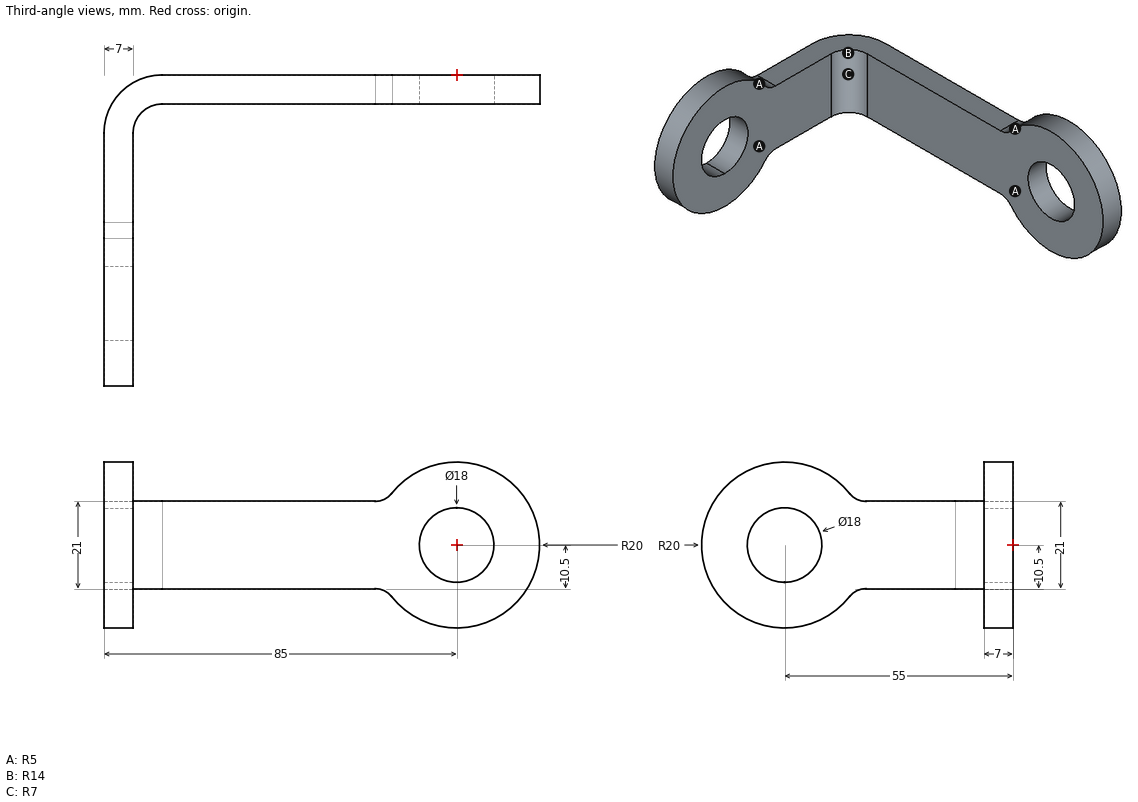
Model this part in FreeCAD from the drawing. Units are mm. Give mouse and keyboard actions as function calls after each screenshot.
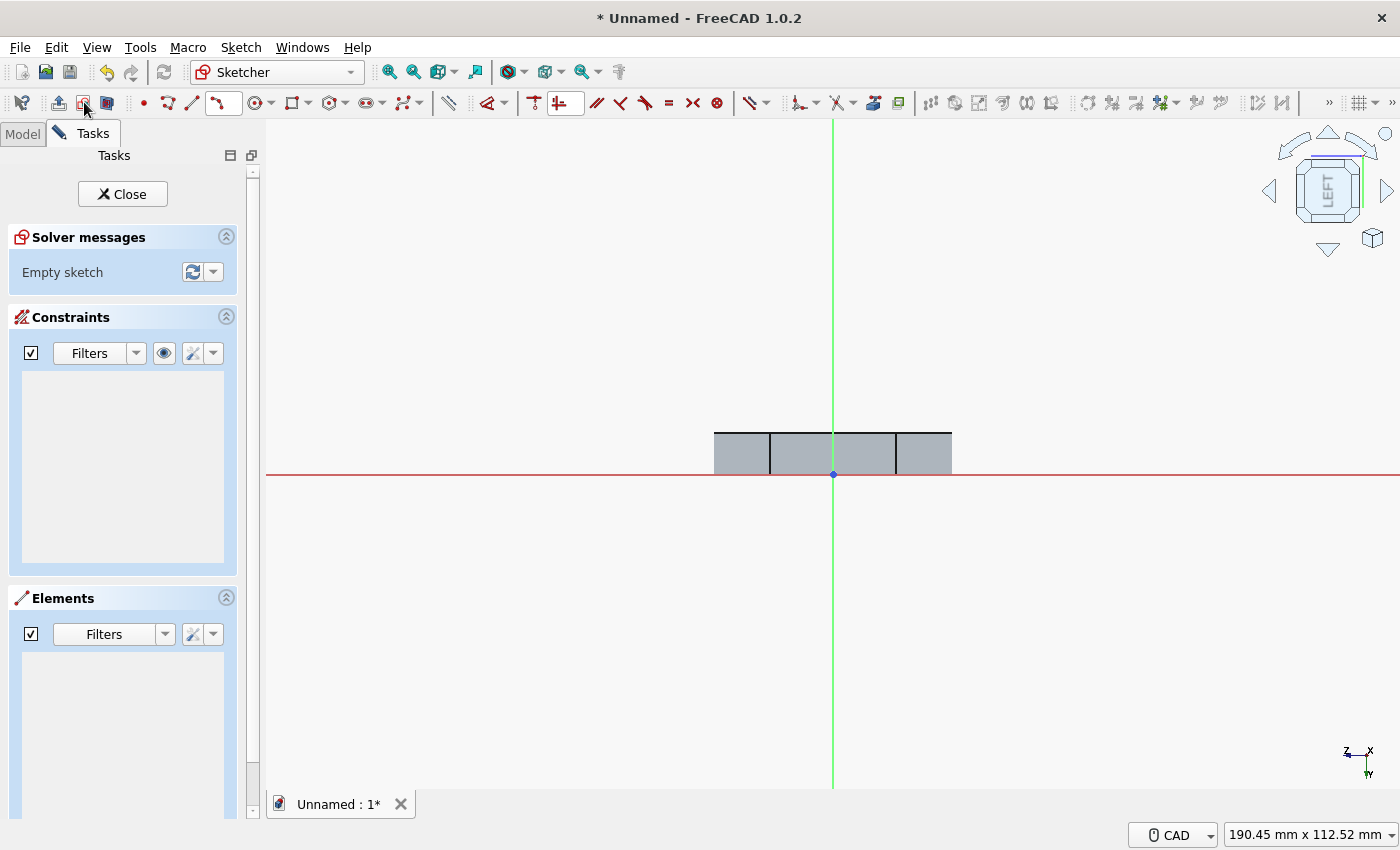
scroll(625, 761, down, 2)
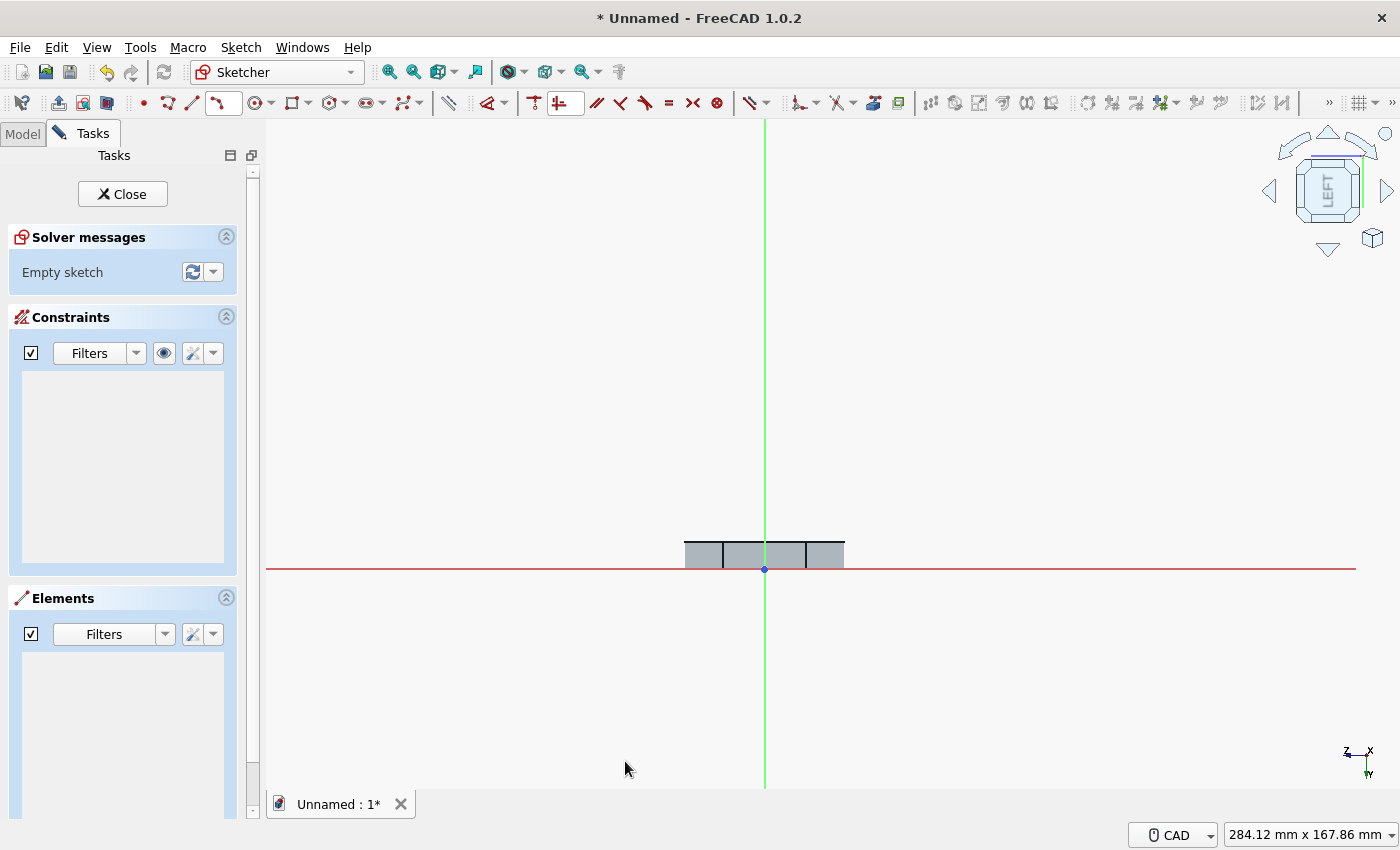
scroll(765, 350, up, 2)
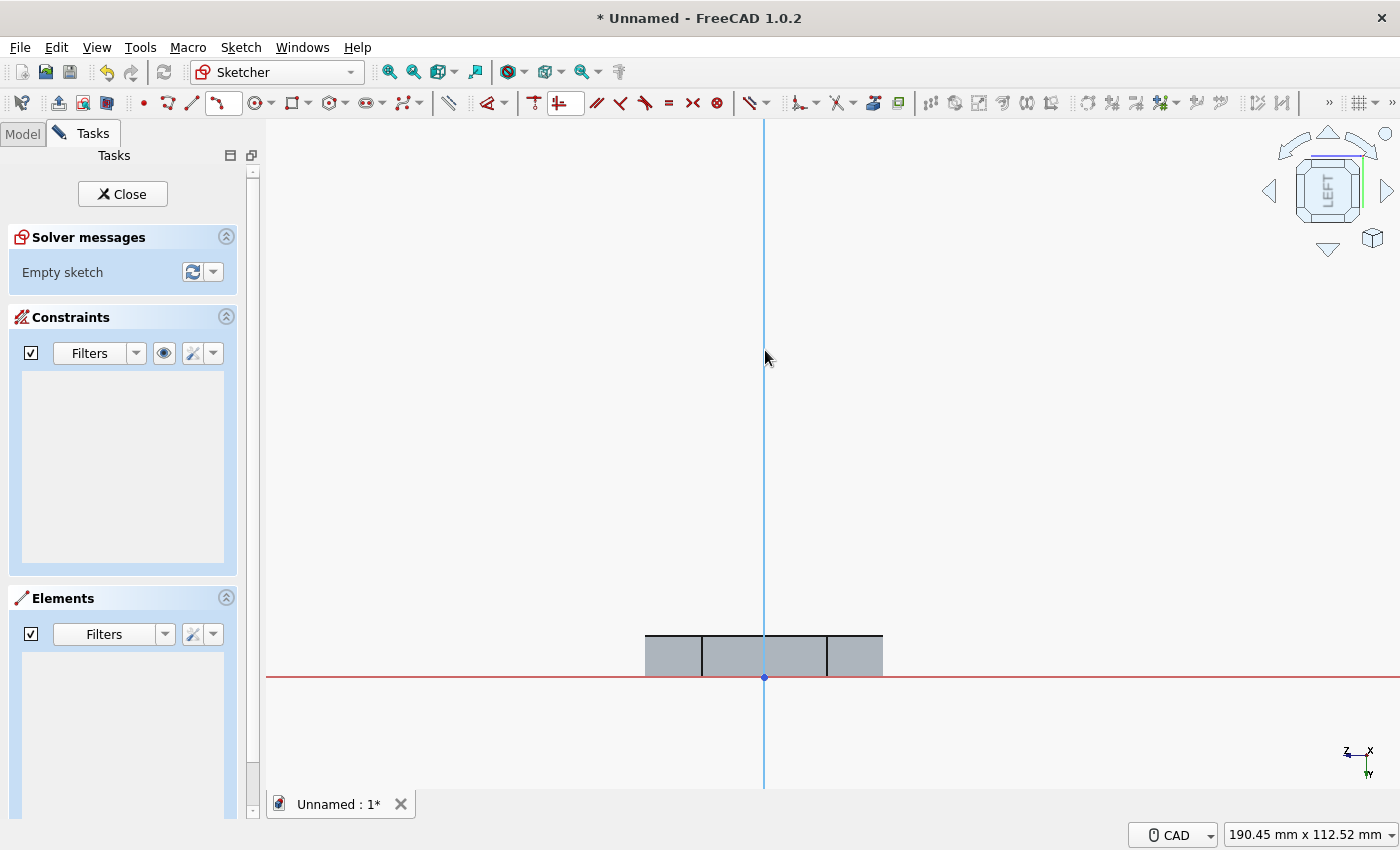
click(168, 104)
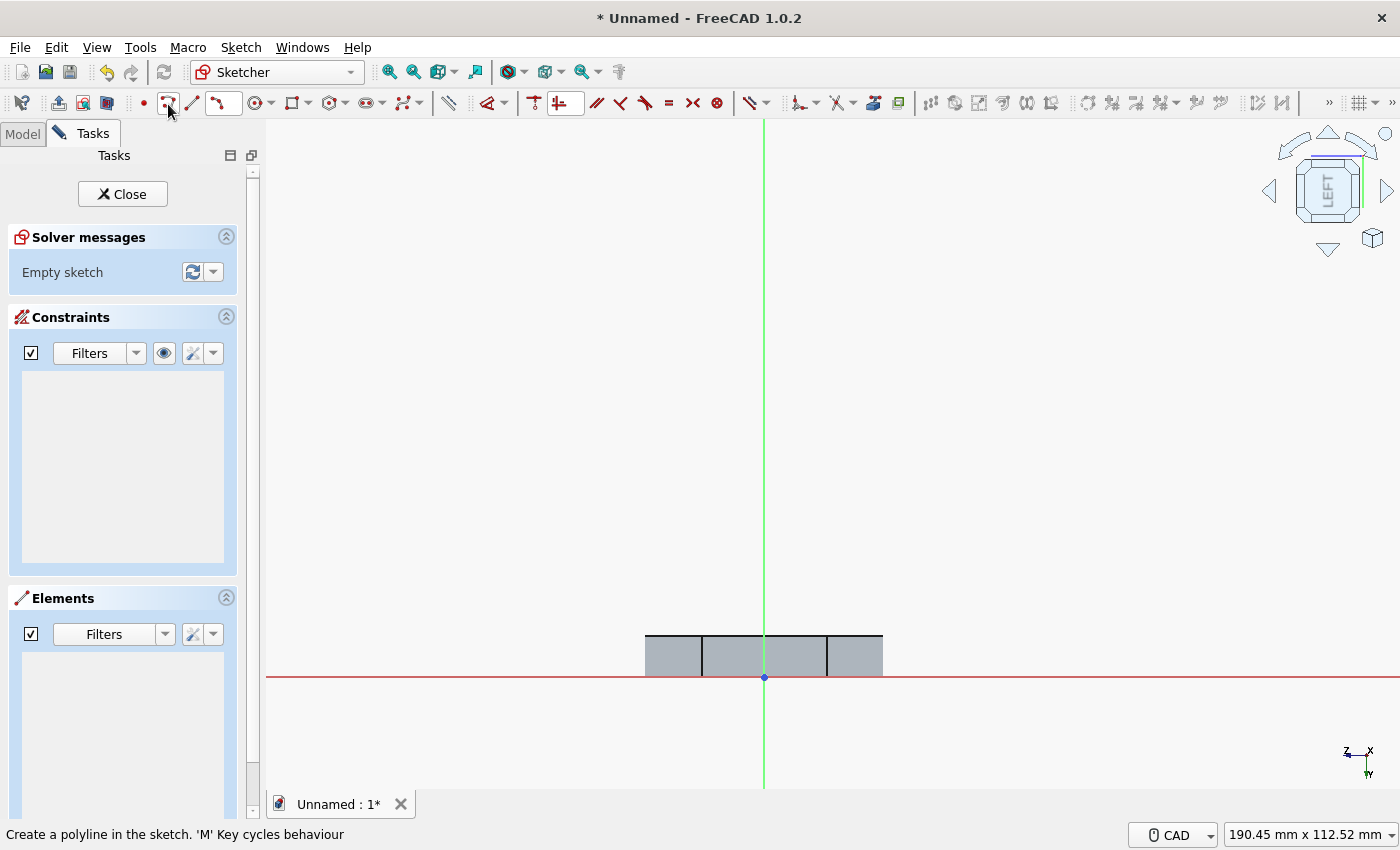
click(827, 451)
click(827, 677)
click(702, 668)
click(702, 451)
right_click(702, 451)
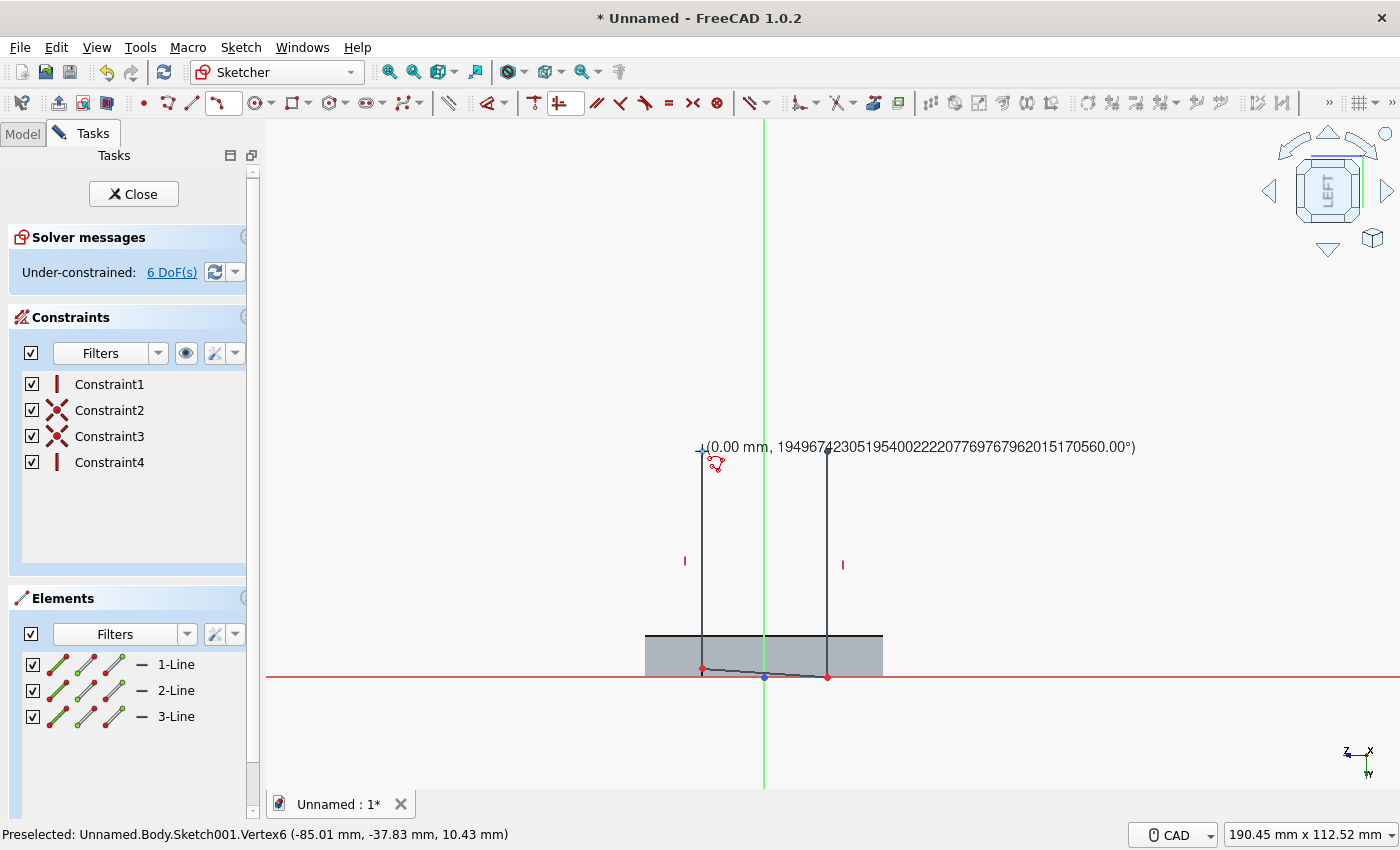
click(218, 104)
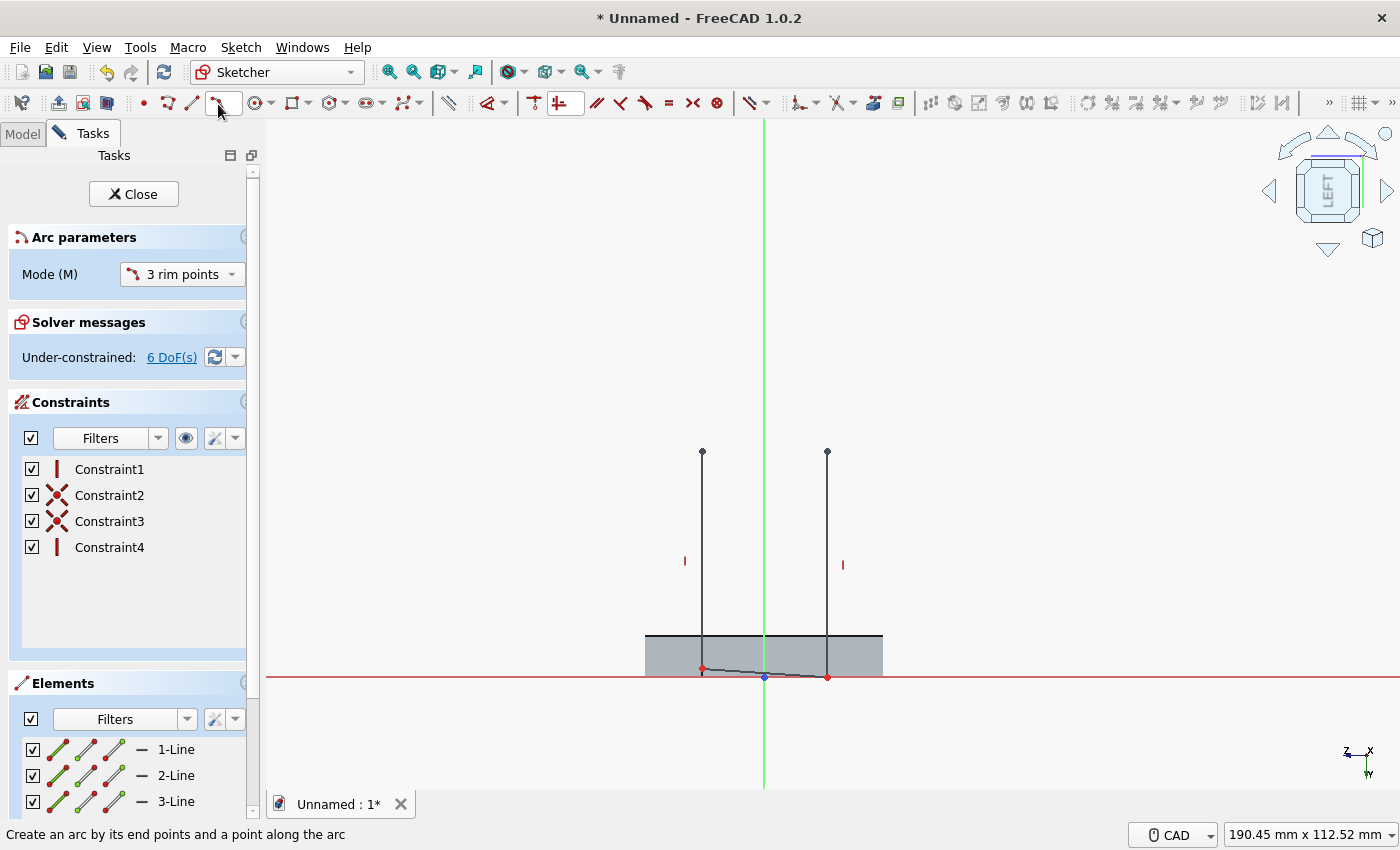
click(702, 452)
click(827, 452)
click(823, 246)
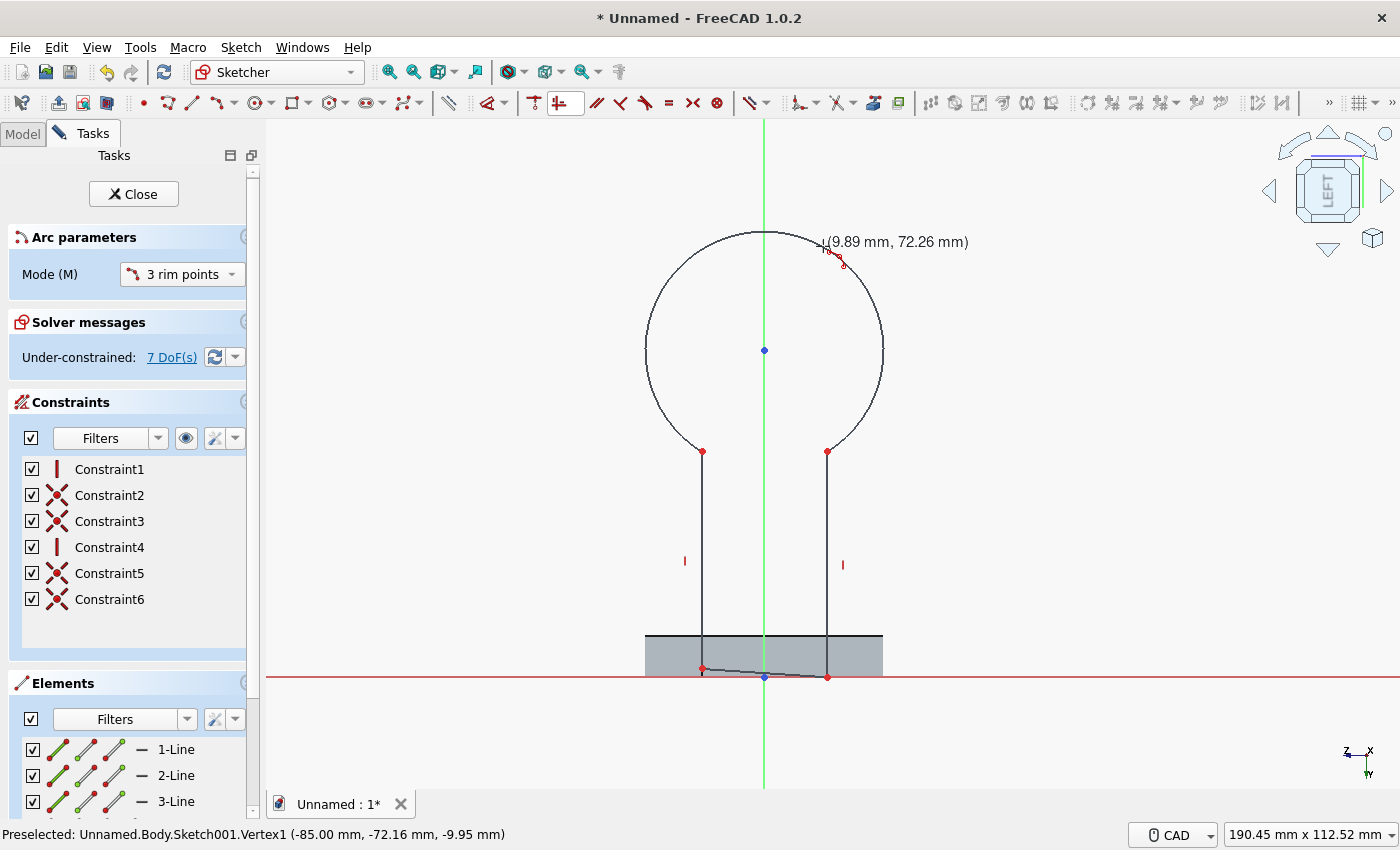
click(256, 104)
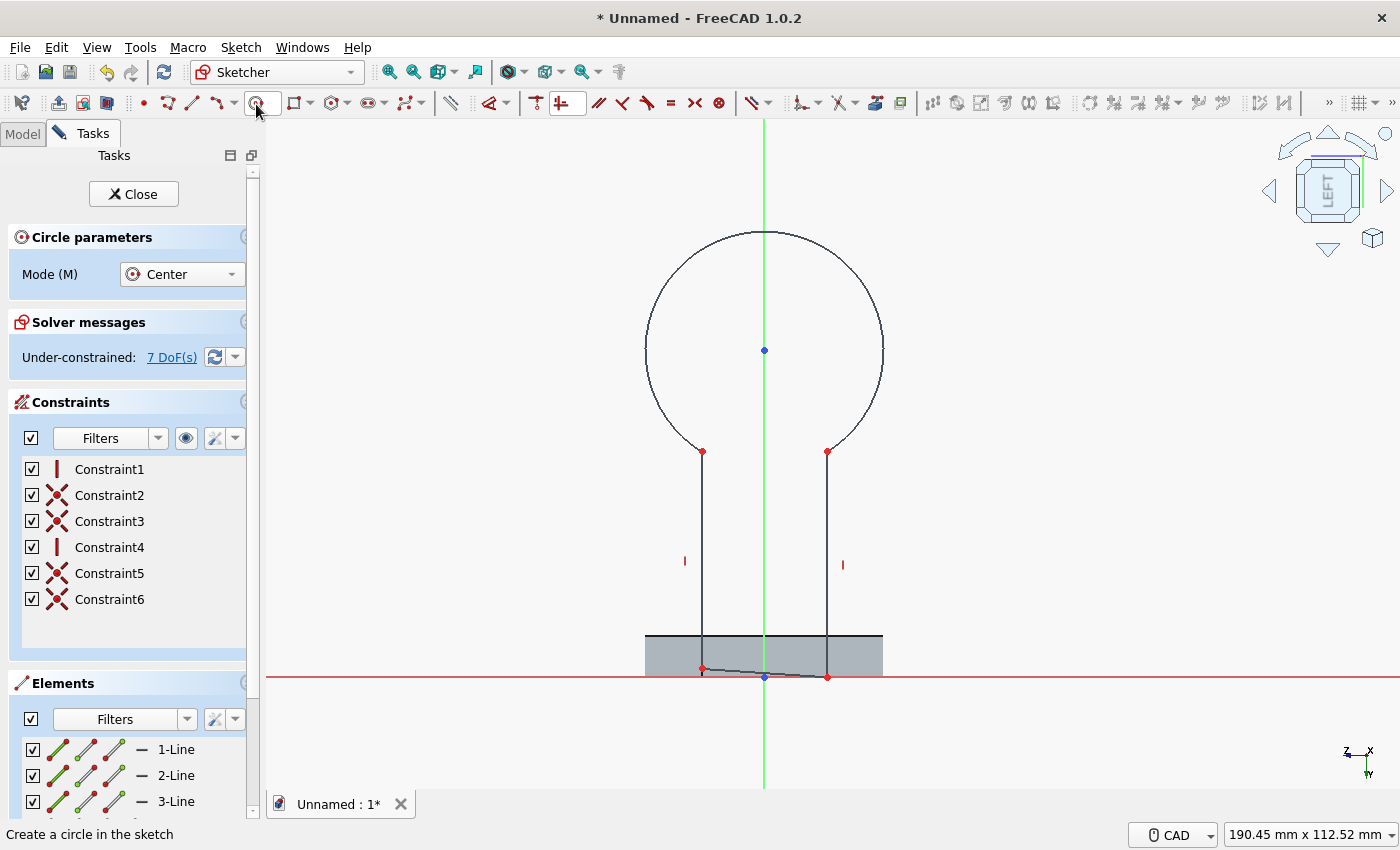
click(764, 350)
move(802, 312)